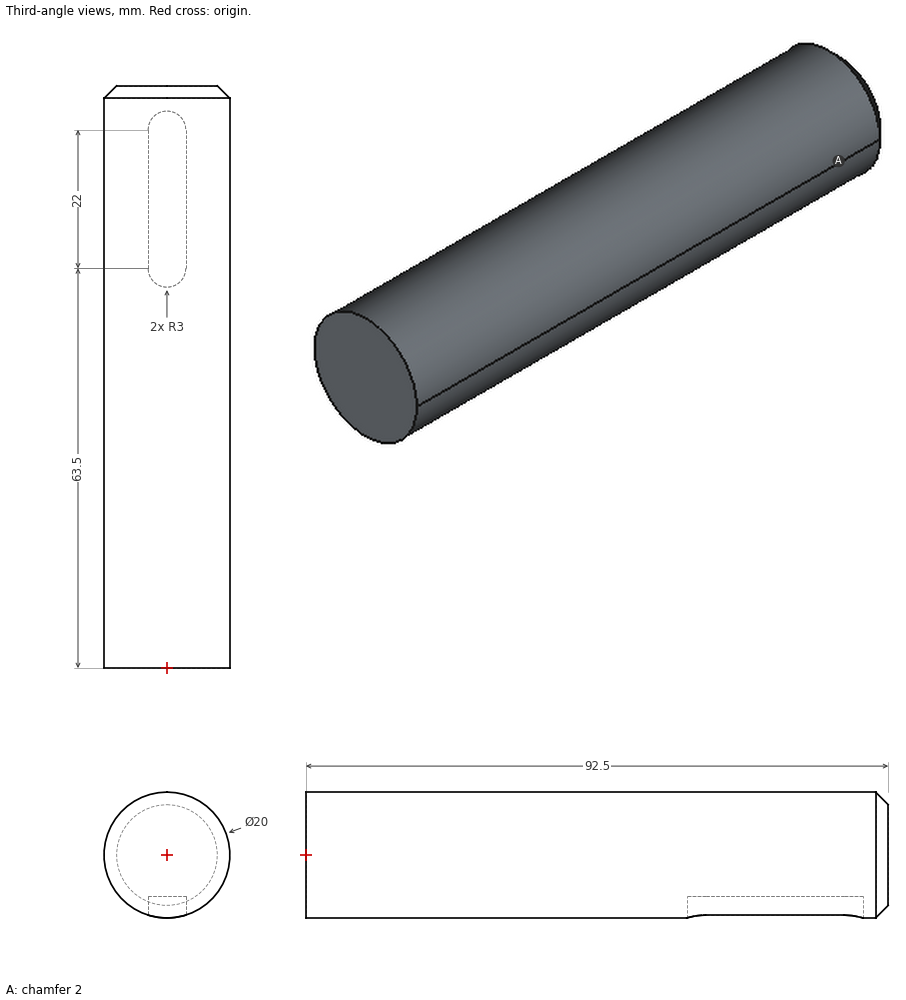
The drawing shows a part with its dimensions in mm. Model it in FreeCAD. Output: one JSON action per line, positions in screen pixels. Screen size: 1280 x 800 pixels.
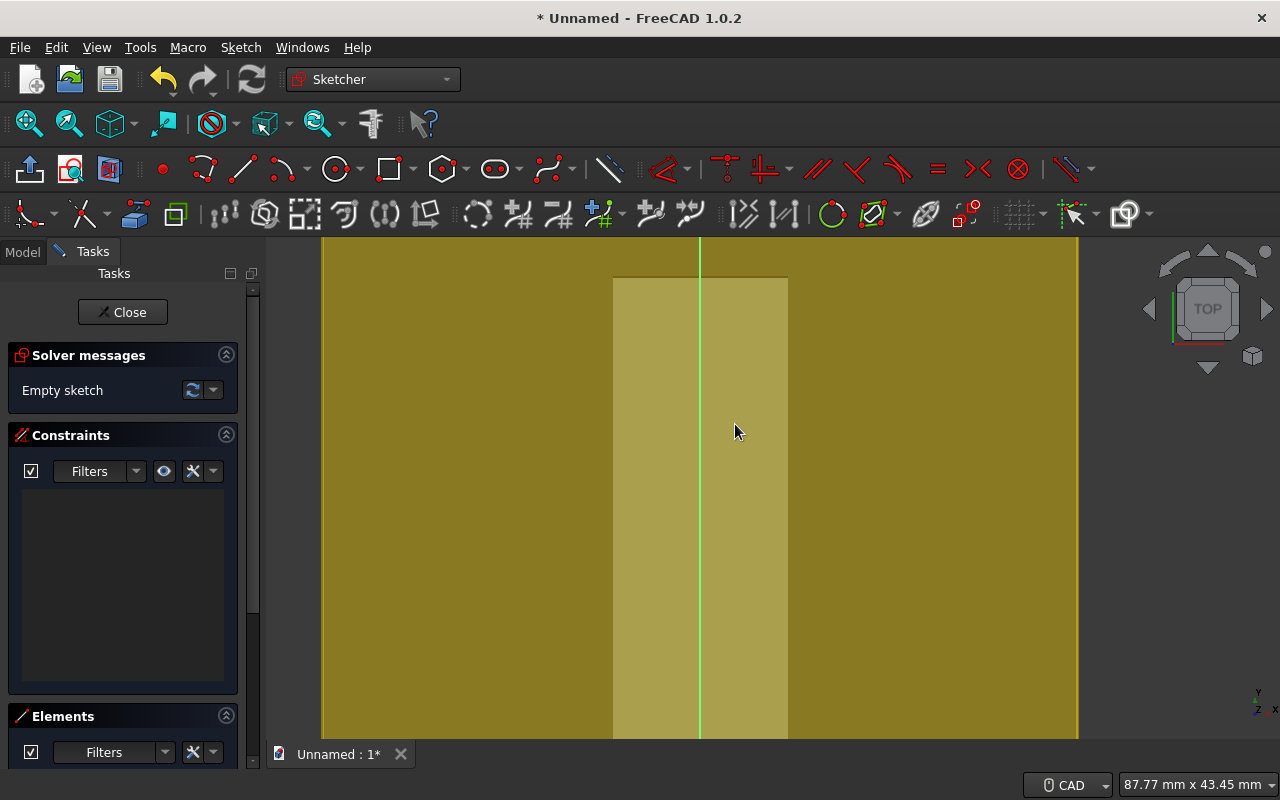
{"action": "key", "text": "g s"}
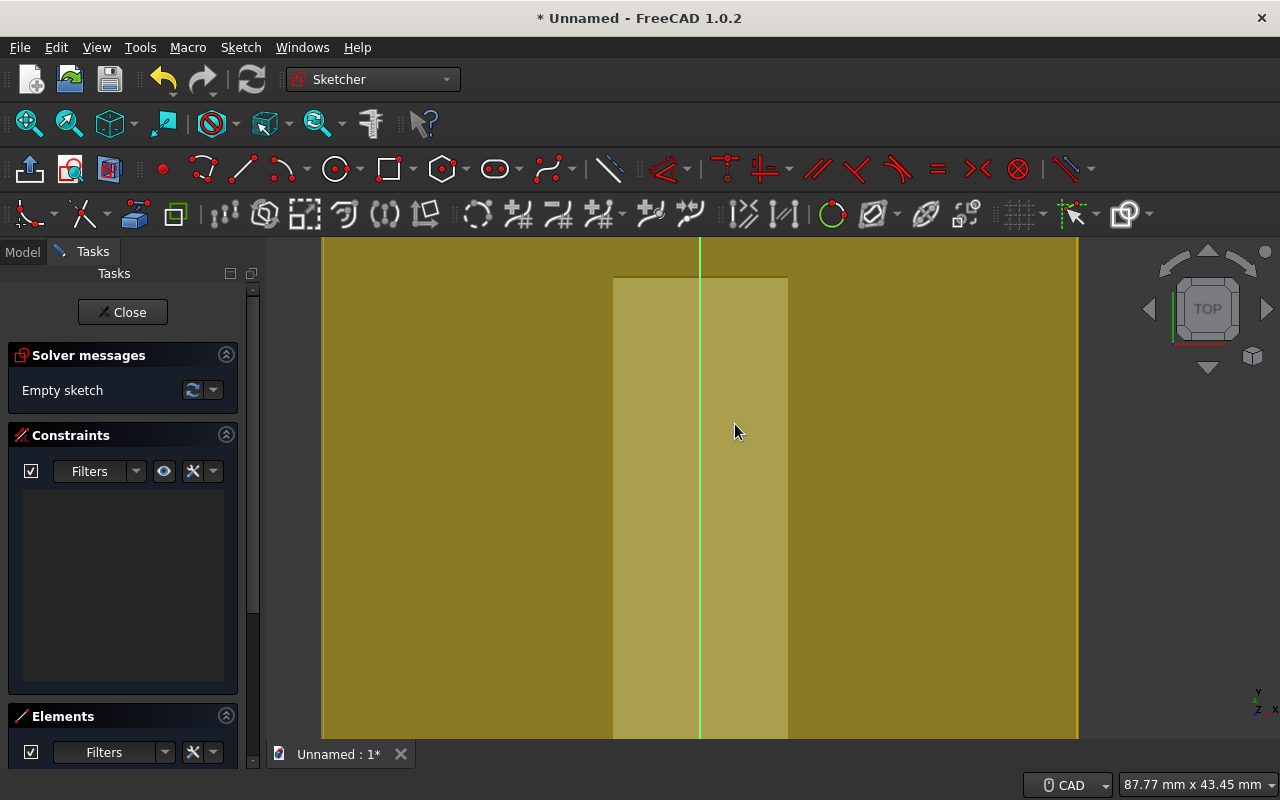
{"action": "left_click", "coordinate": [700, 612]}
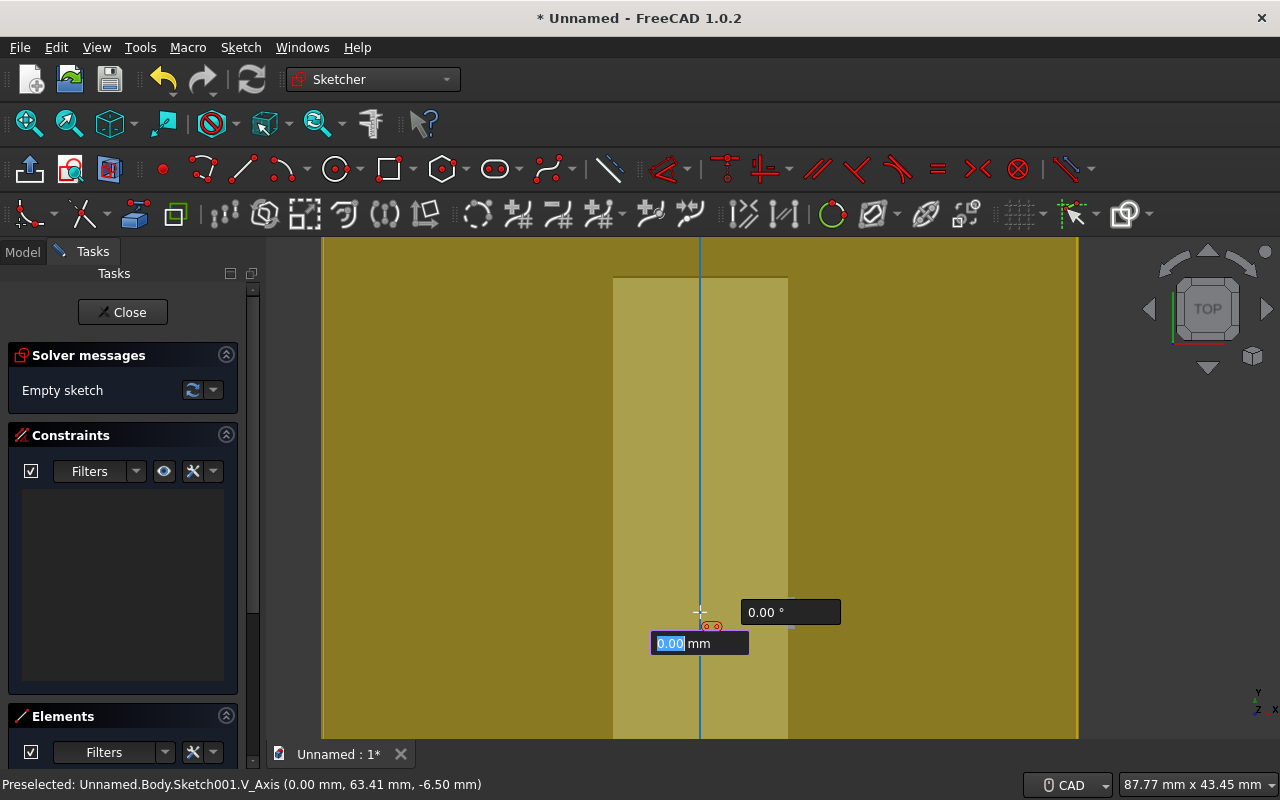
{"action": "left_click", "coordinate": [709, 358]}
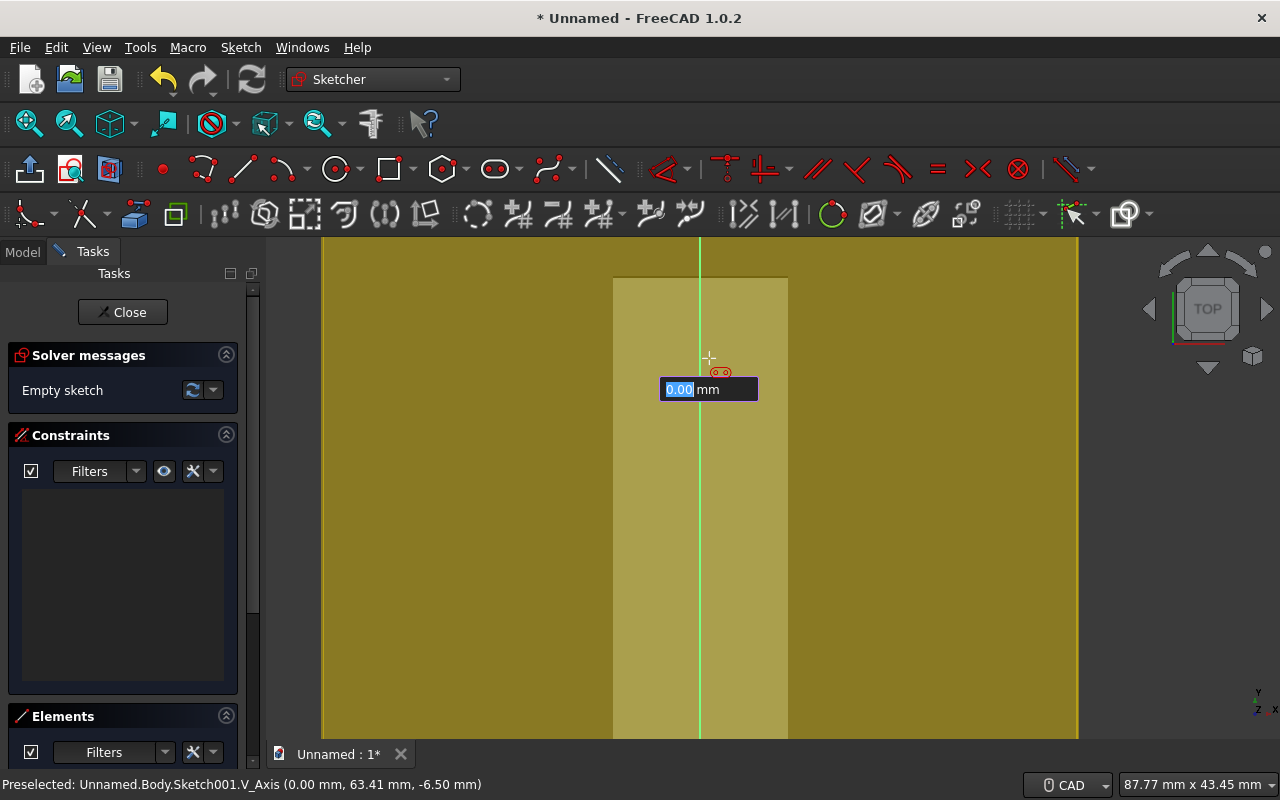
{"action": "left_click", "coordinate": [666, 485]}
{"action": "key", "text": "Escape"}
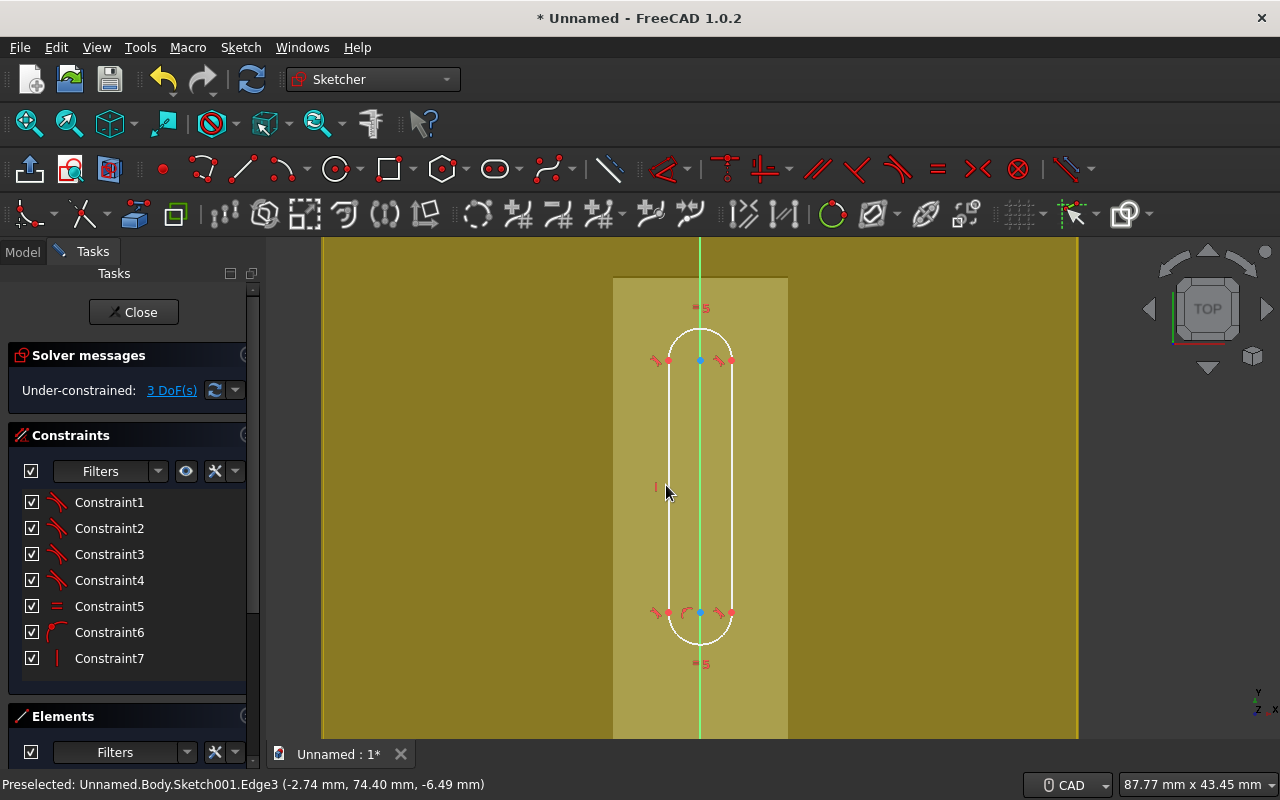
{"action": "left_click", "coordinate": [664, 170]}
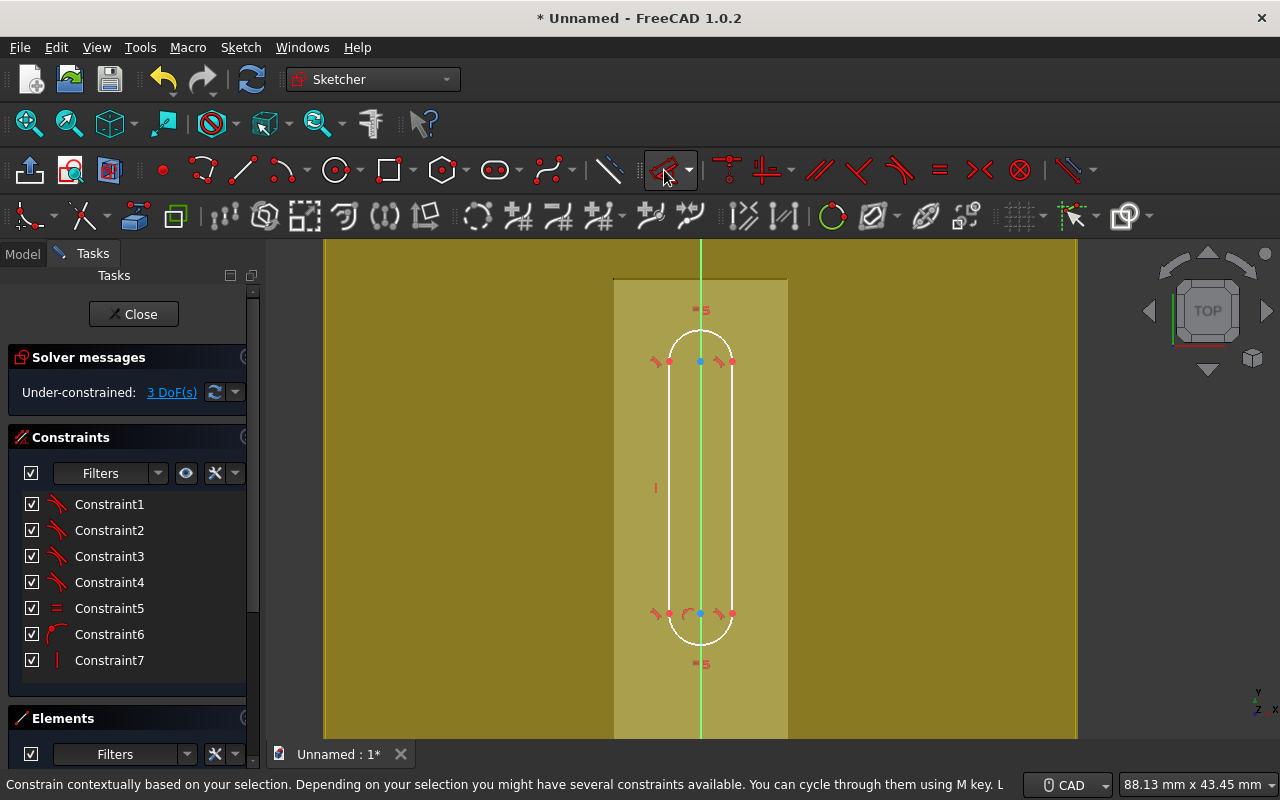
{"action": "left_click", "coordinate": [682, 639]}
{"action": "left_click", "coordinate": [663, 665]}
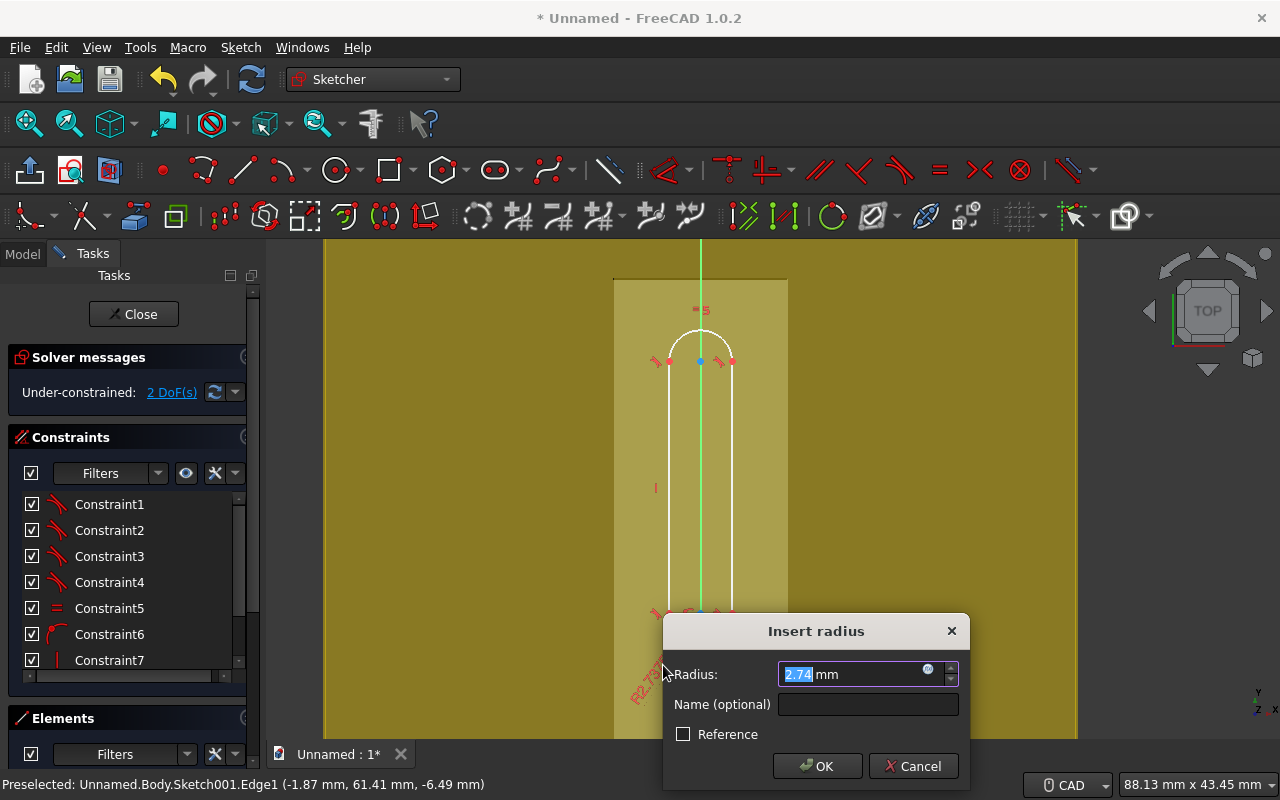
{"action": "type", "text": "3"}
{"action": "key", "text": "Return"}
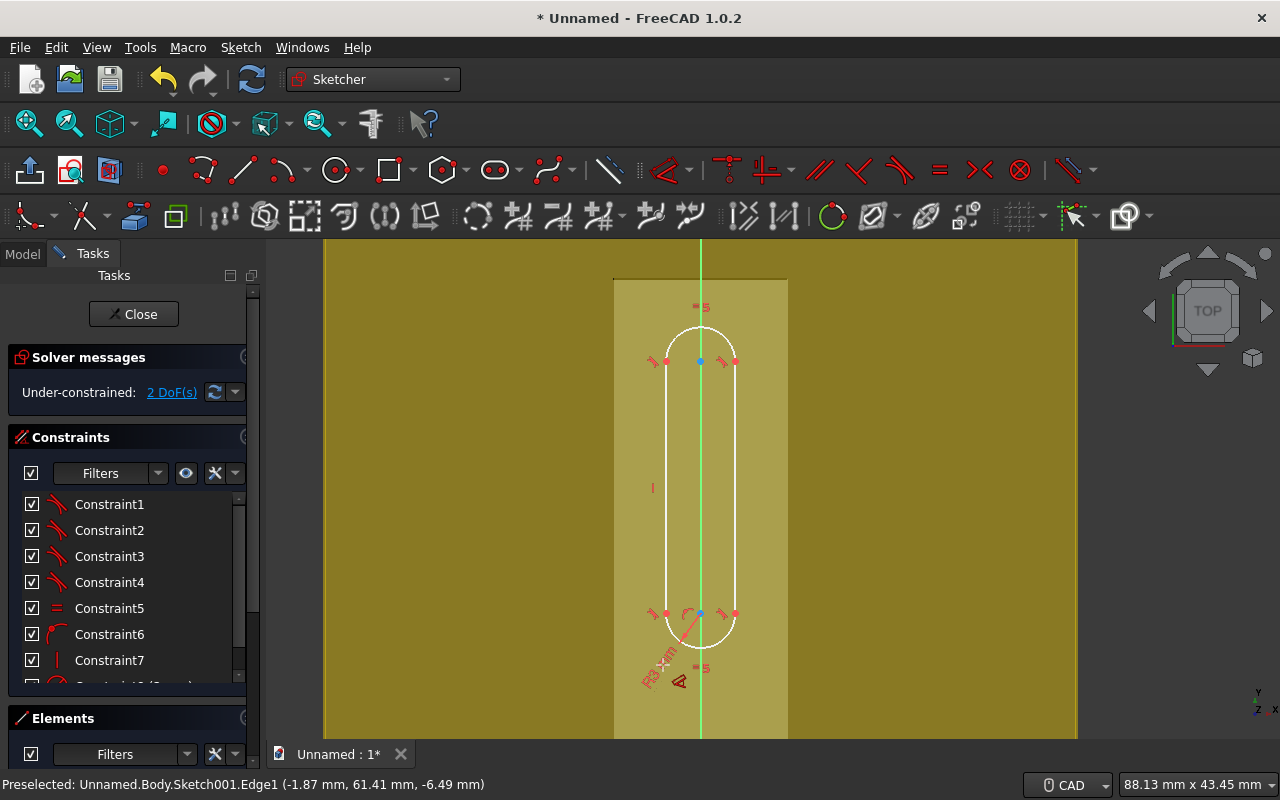
{"action": "left_click", "coordinate": [666, 538]}
{"action": "left_click", "coordinate": [632, 488]}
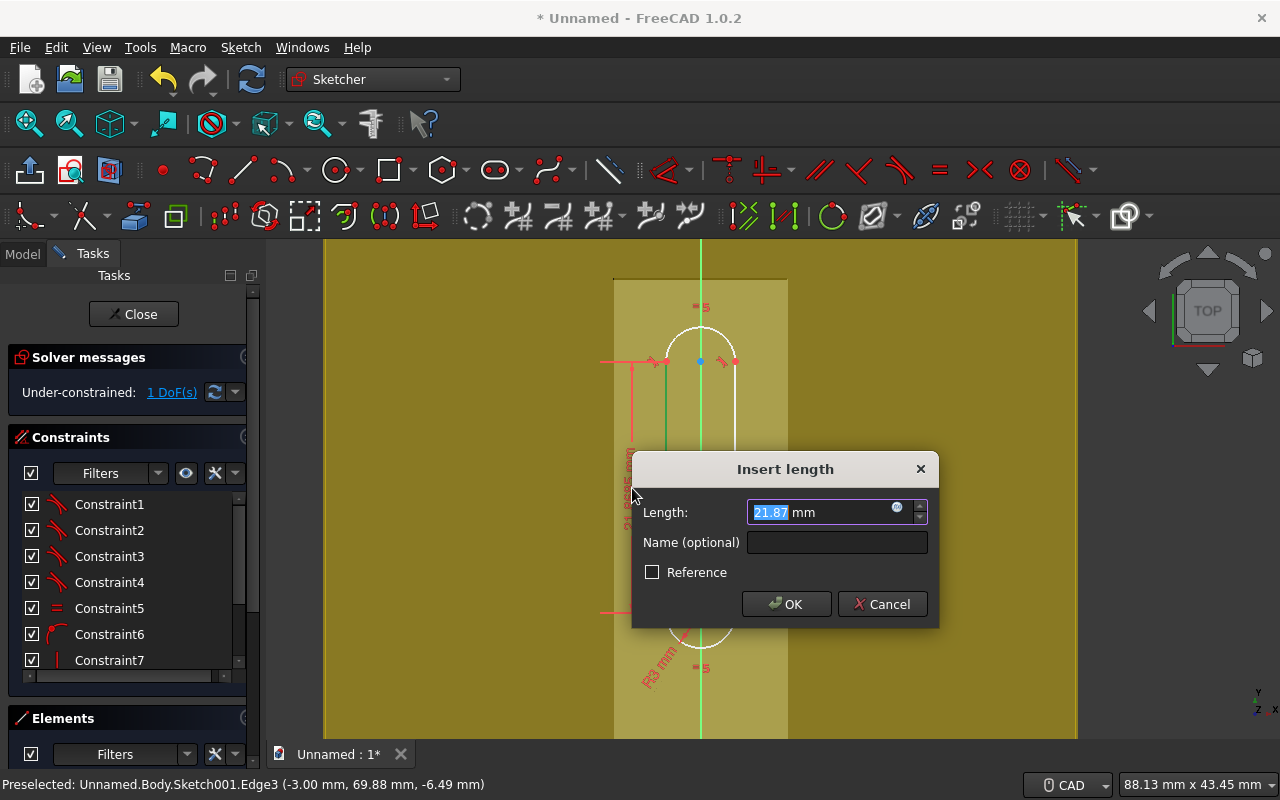
{"action": "type", "text": "22"}
{"action": "key", "text": "Return"}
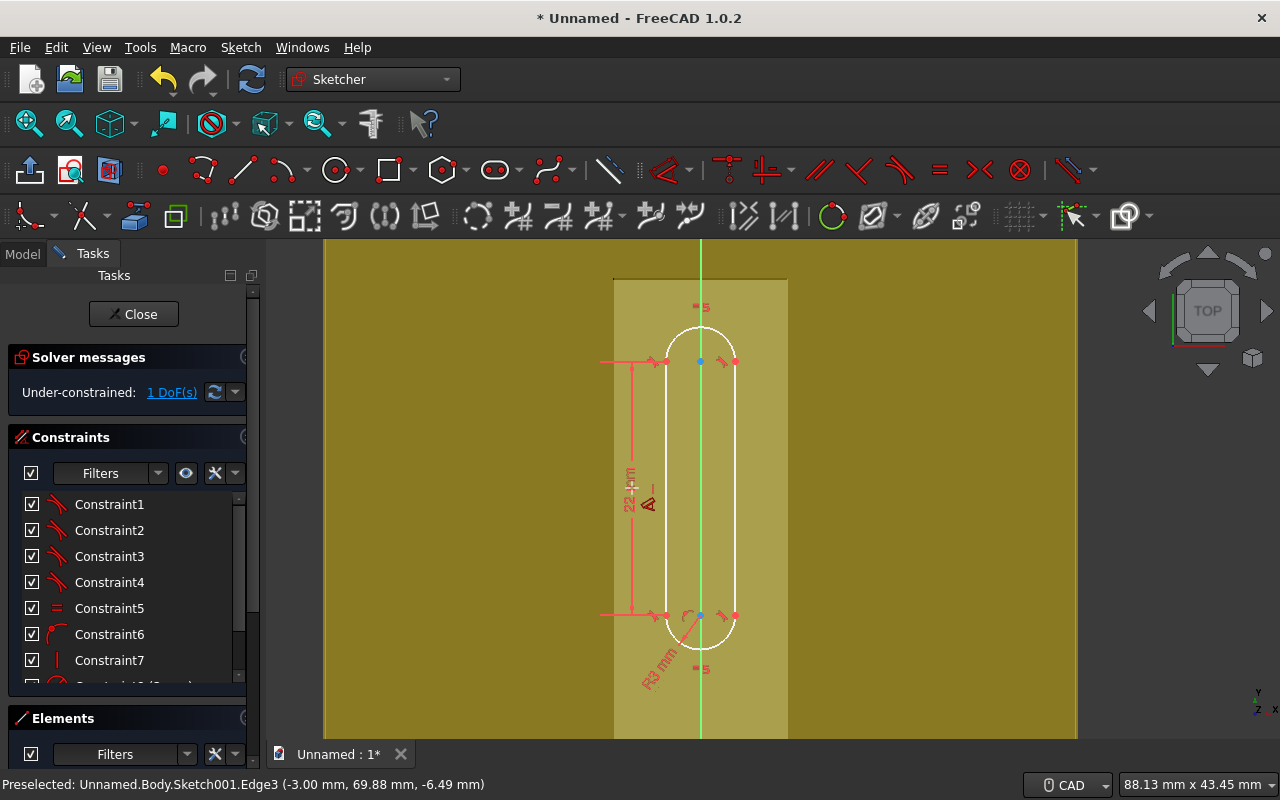
{"action": "left_click", "coordinate": [666, 615]}
{"action": "left_click", "coordinate": [632, 641]}